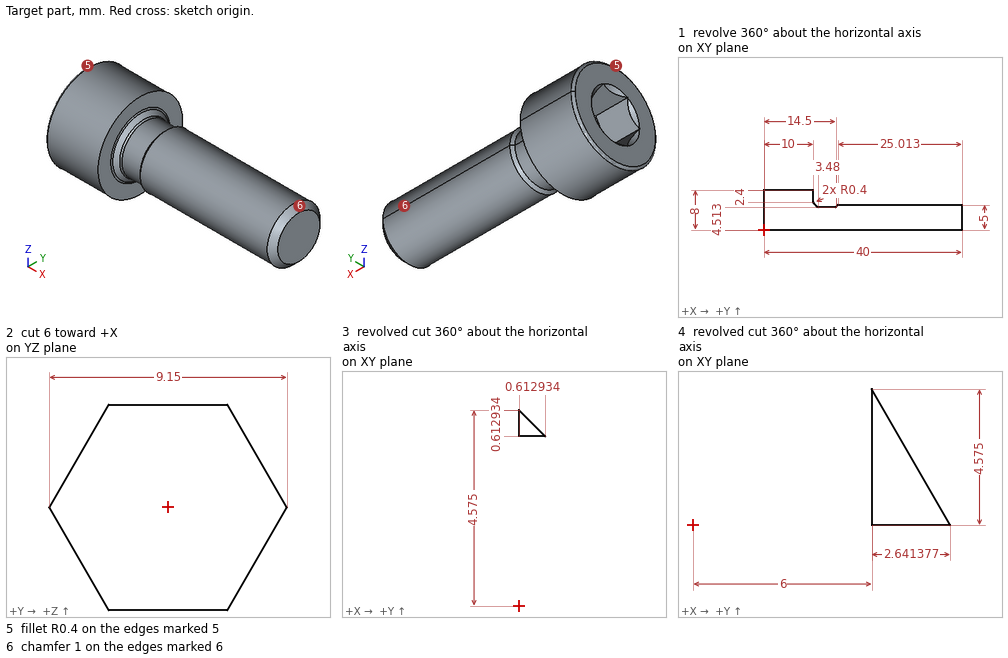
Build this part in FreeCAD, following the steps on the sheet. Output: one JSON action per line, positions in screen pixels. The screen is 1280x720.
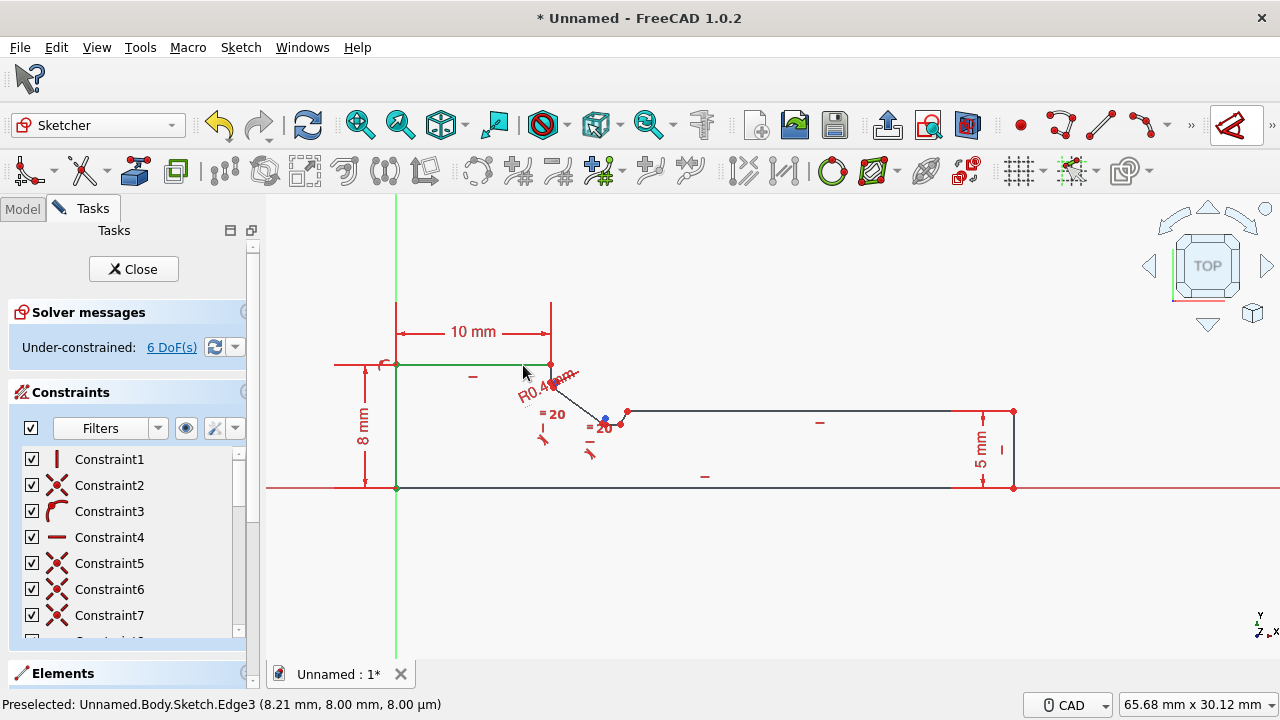
{"action": "left_click", "coordinate": [582, 488]}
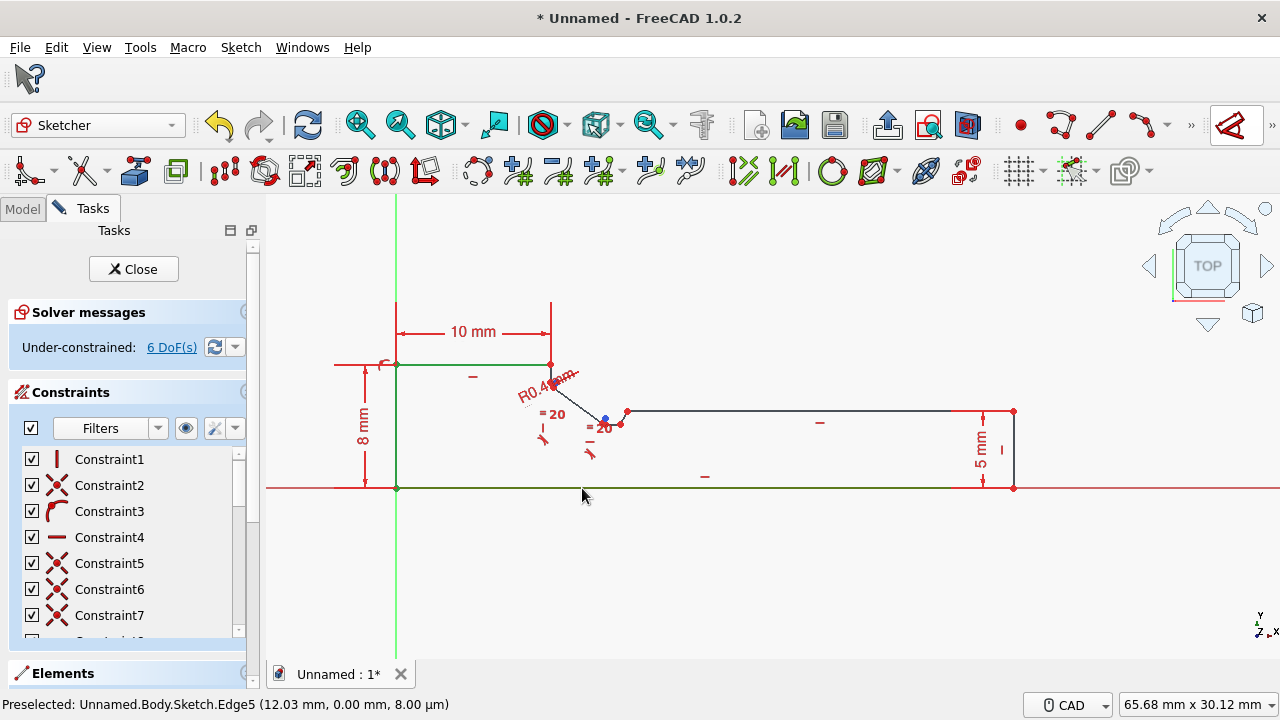
{"action": "left_click", "coordinate": [1258, 126]}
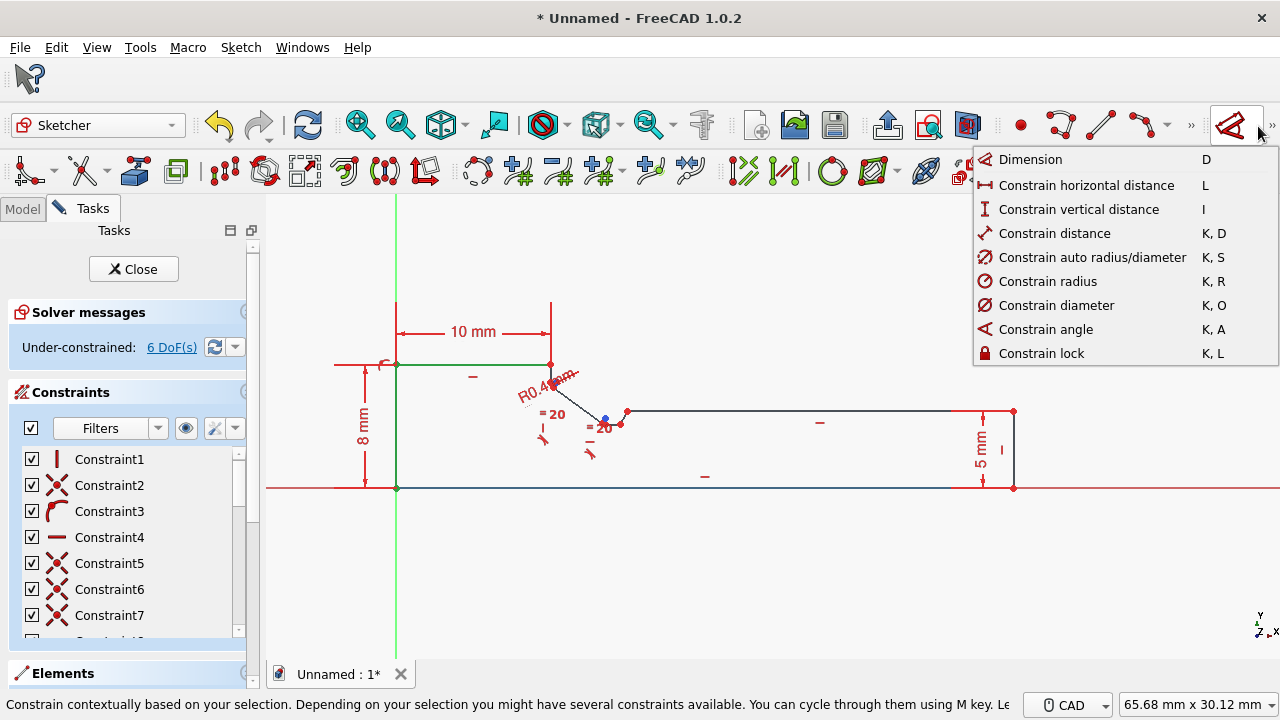
{"action": "left_click", "coordinate": [1126, 185]}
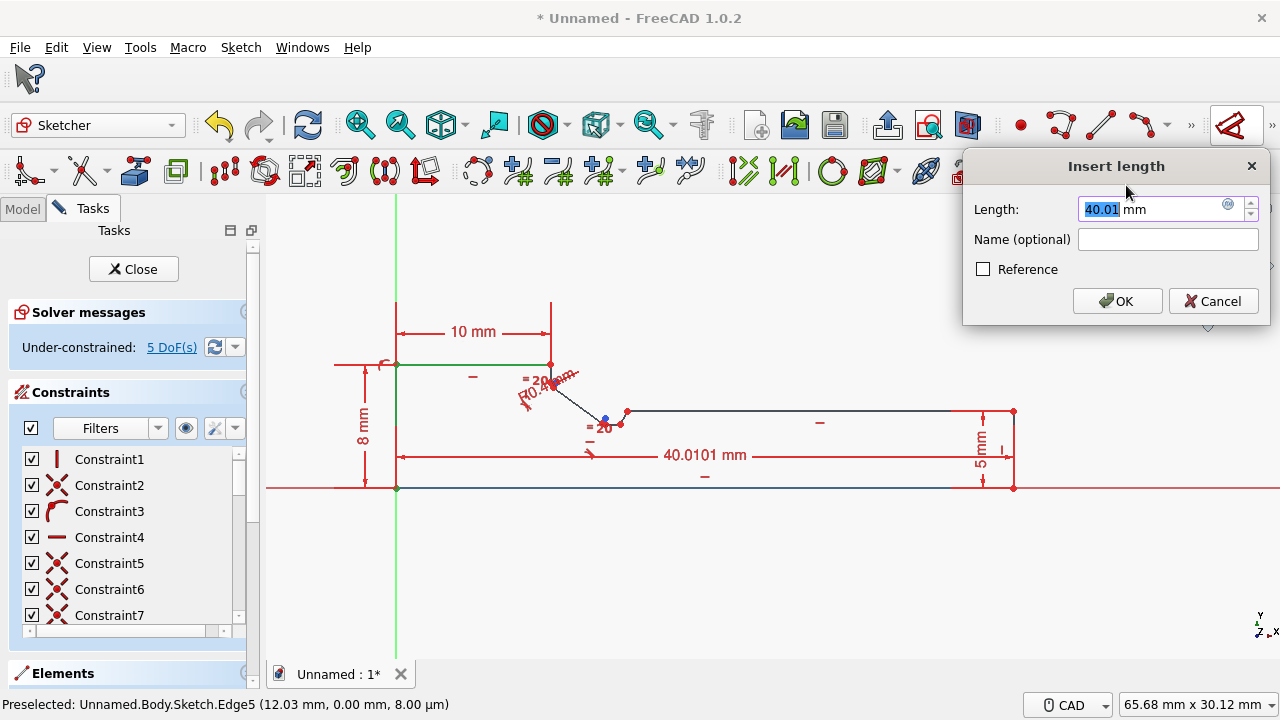
{"action": "type", "text": "40"}
{"action": "key", "text": "Return"}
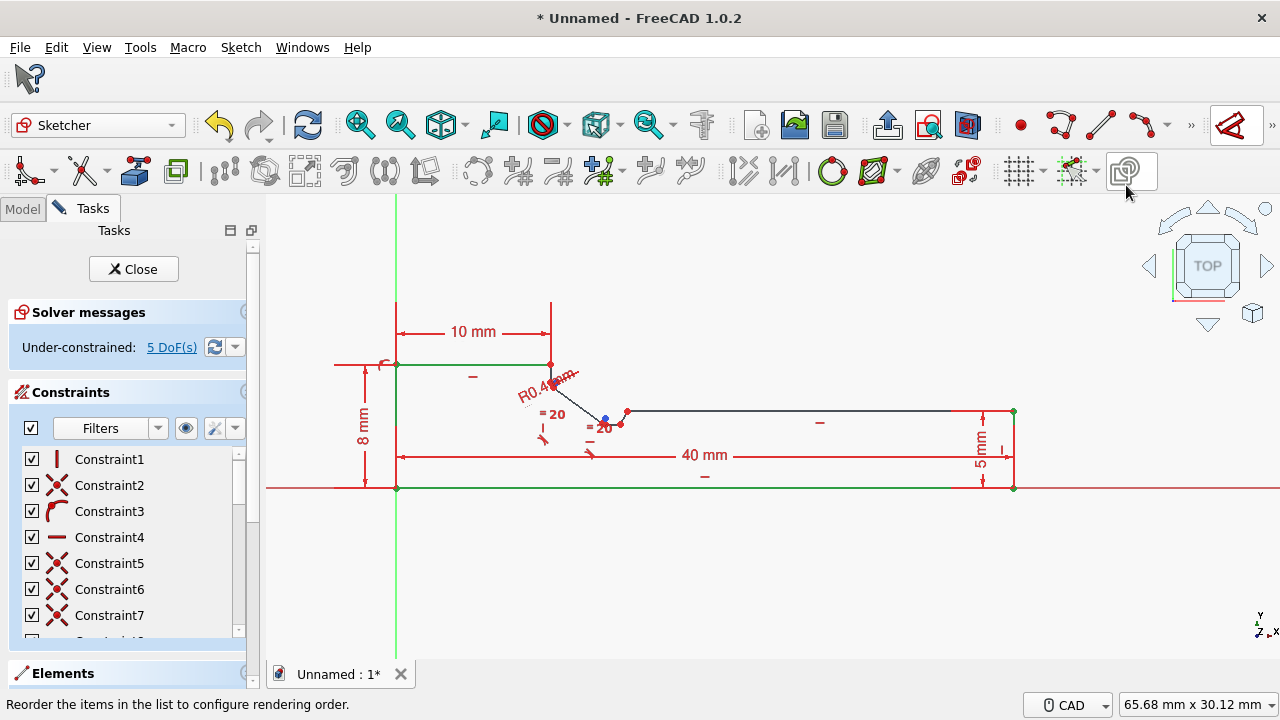
{"action": "scroll", "coordinate": [551, 374], "scroll_direction": "up", "scroll_amount": 3}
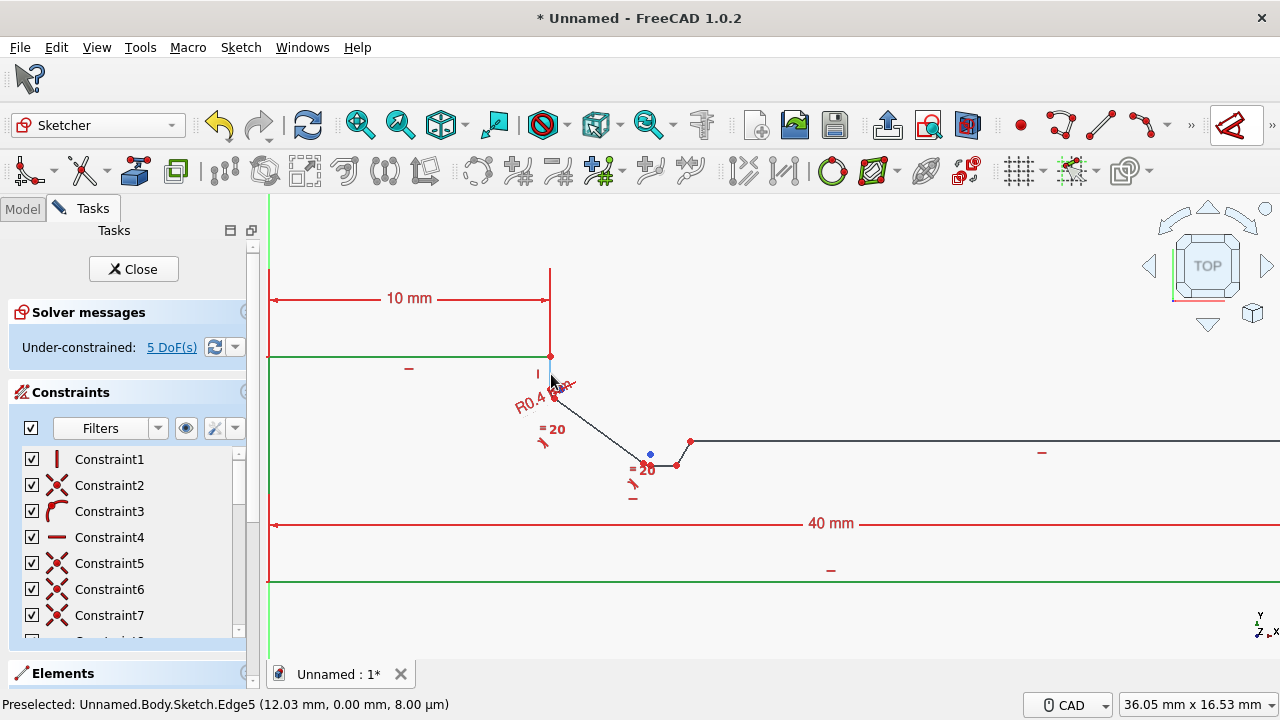
{"action": "left_click", "coordinate": [550, 373]}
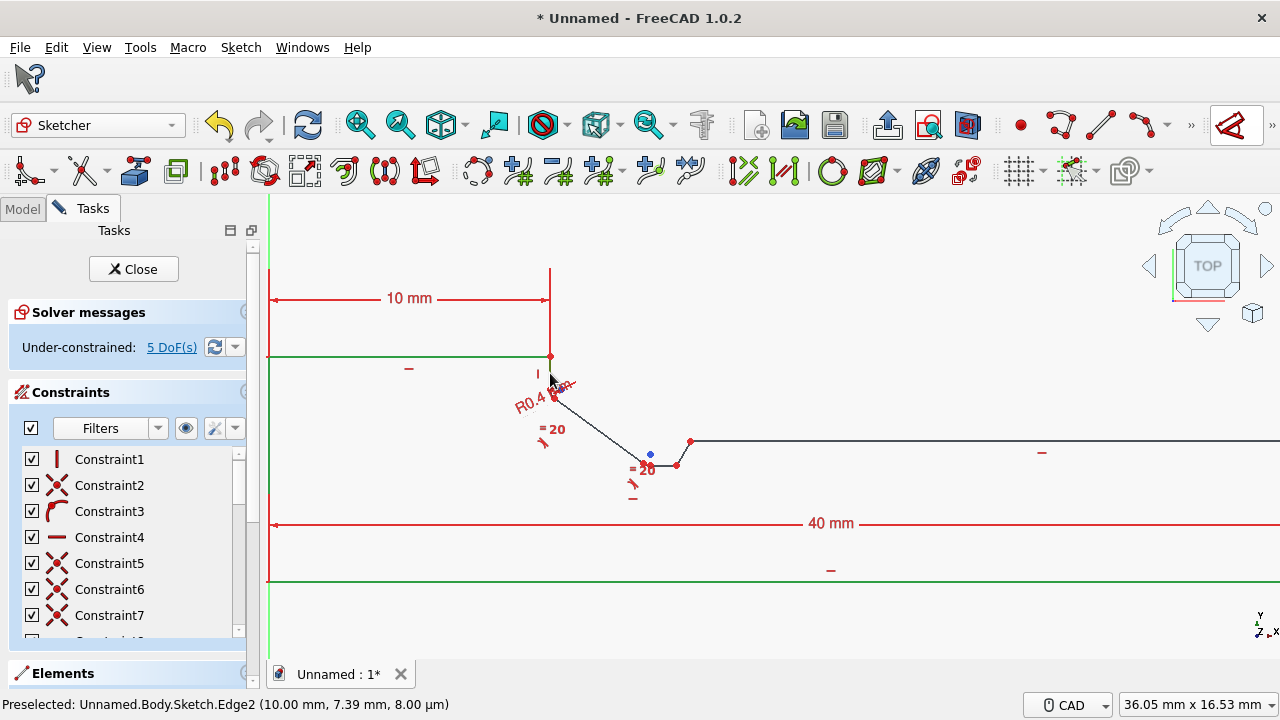
{"action": "key", "text": "i"}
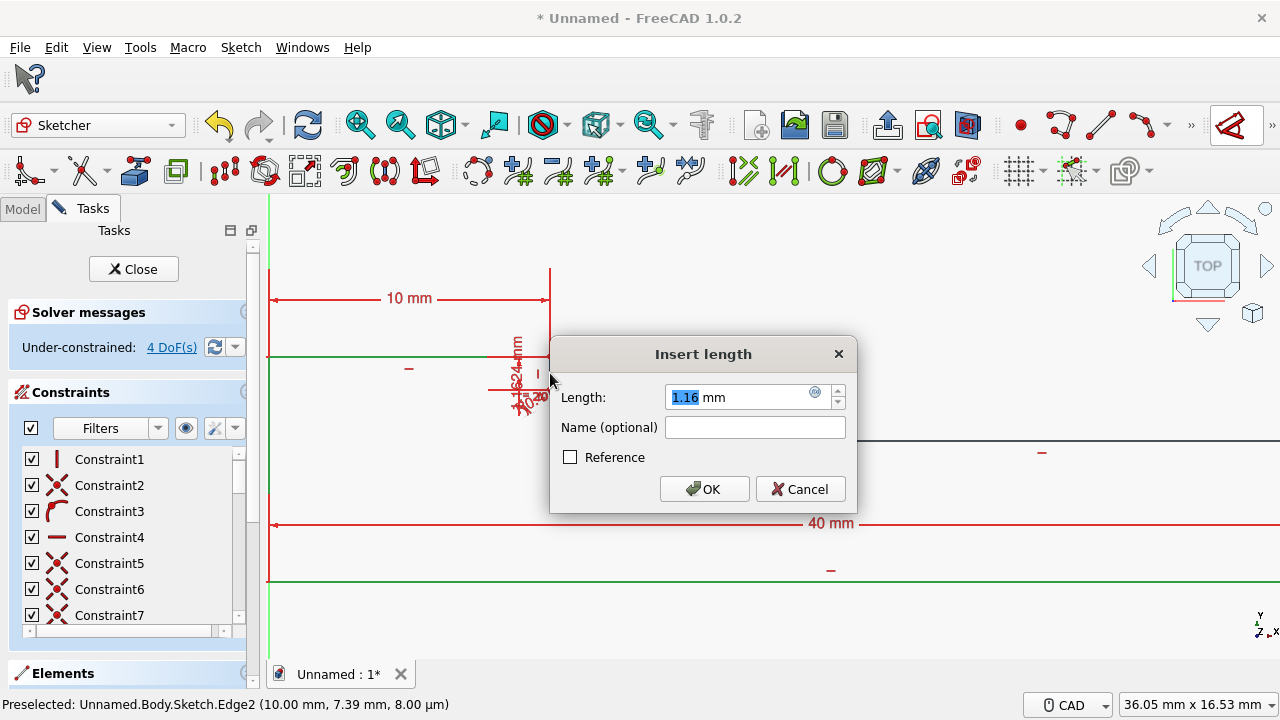
{"action": "type", "text": "2.4"}
{"action": "key", "text": "Return"}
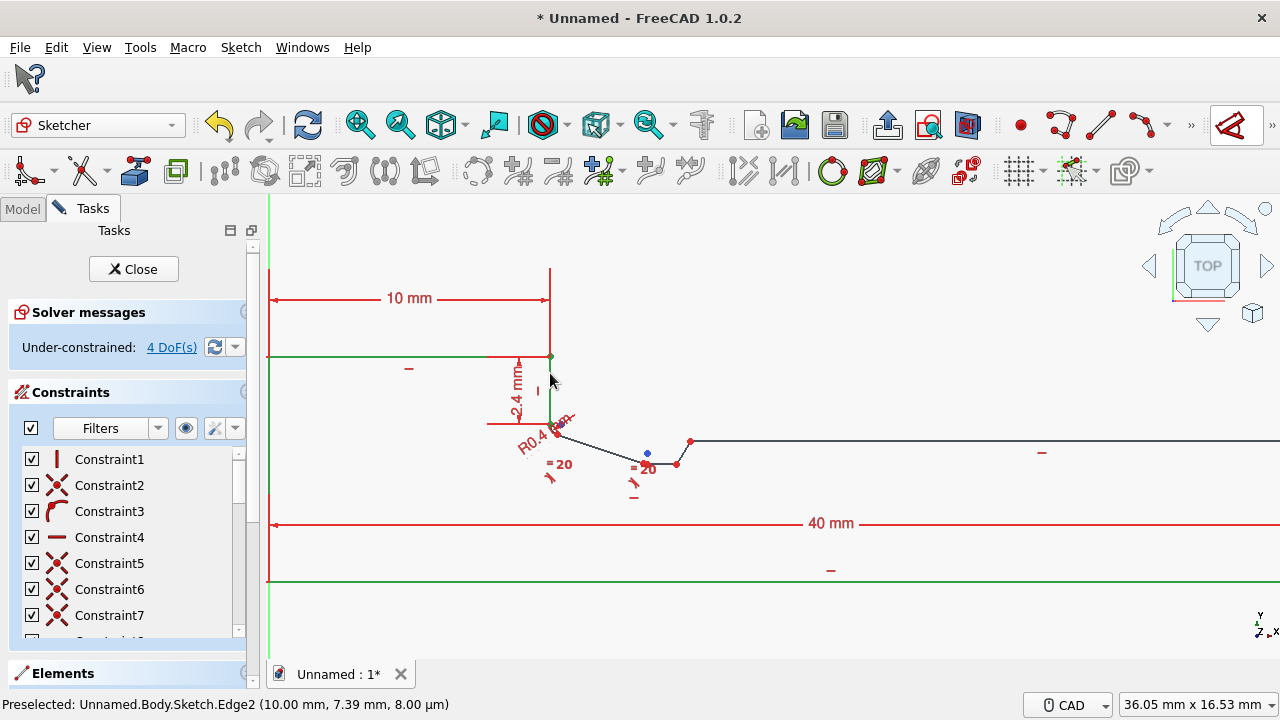
{"action": "left_click", "coordinate": [665, 464]}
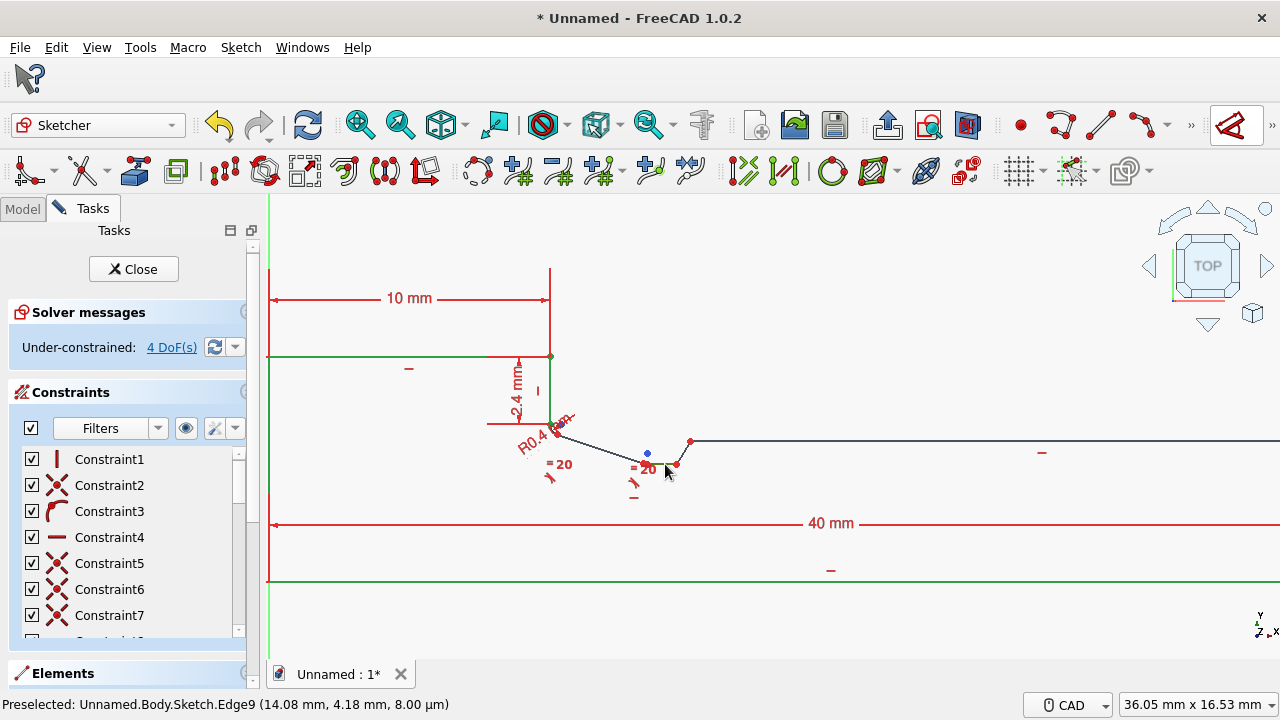
{"action": "key", "text": "l"}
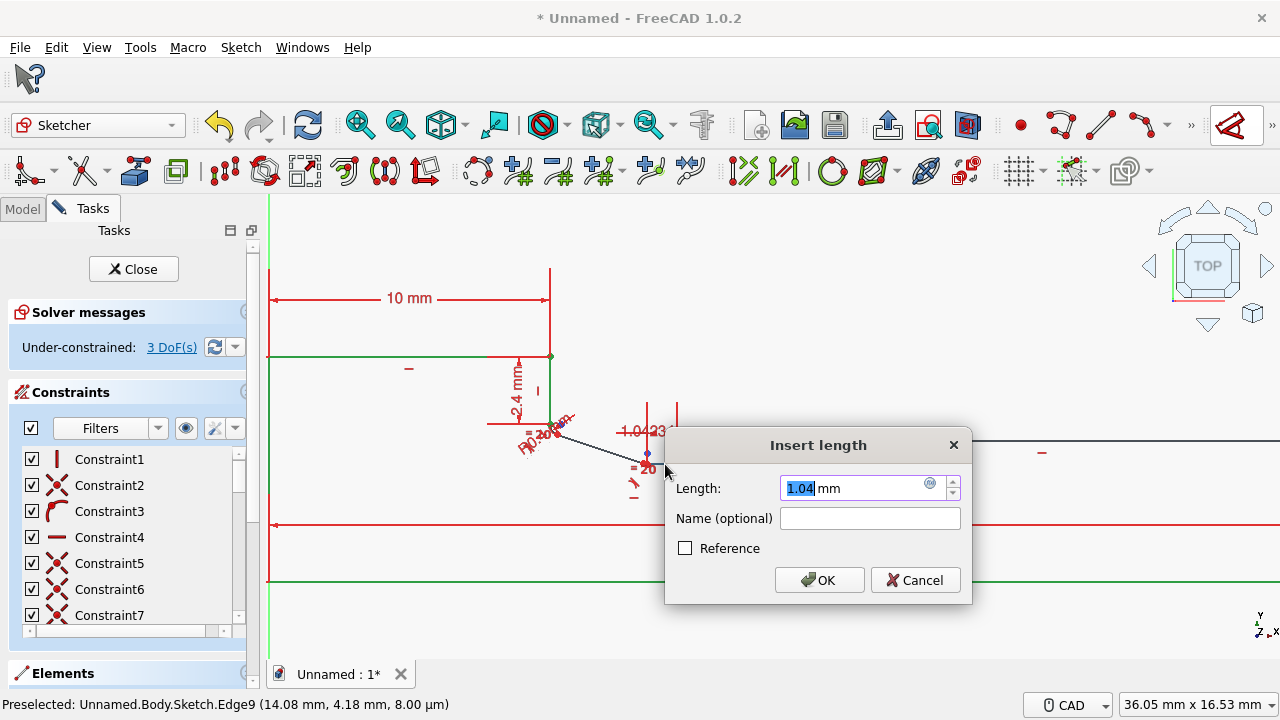
{"action": "type", "text": "3.48"}
{"action": "key", "text": "Return"}